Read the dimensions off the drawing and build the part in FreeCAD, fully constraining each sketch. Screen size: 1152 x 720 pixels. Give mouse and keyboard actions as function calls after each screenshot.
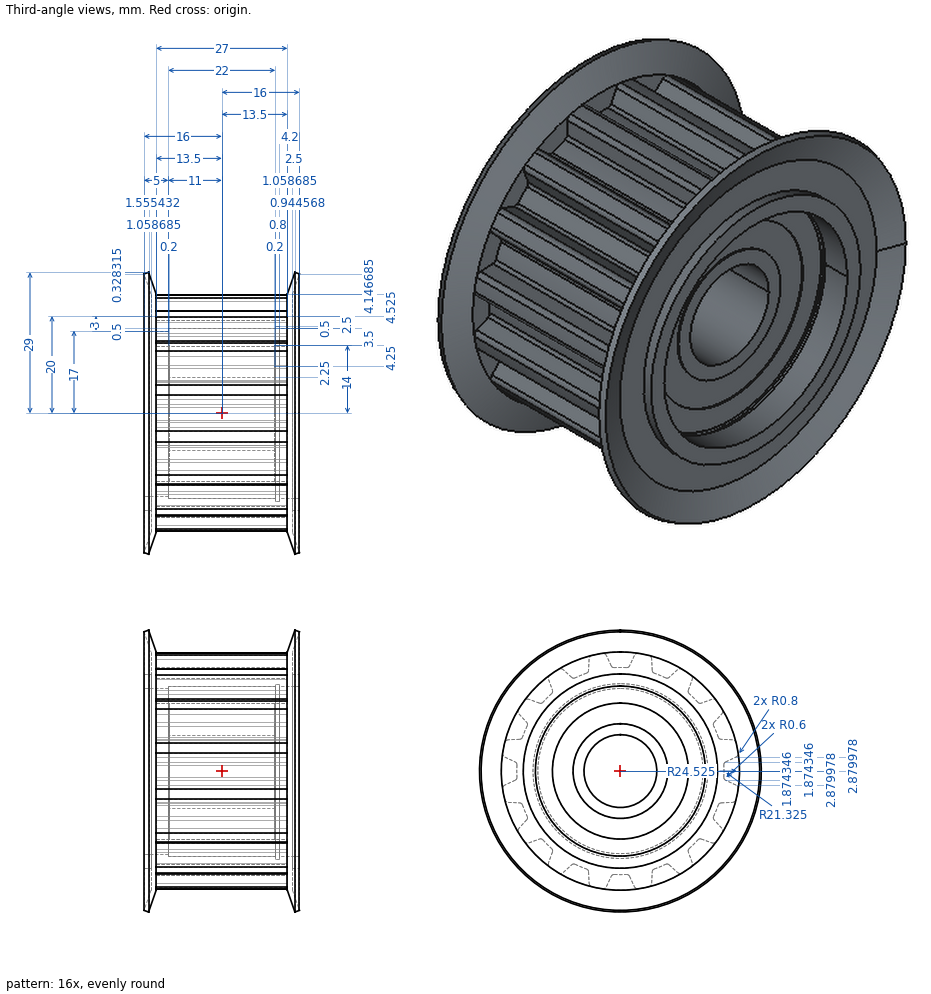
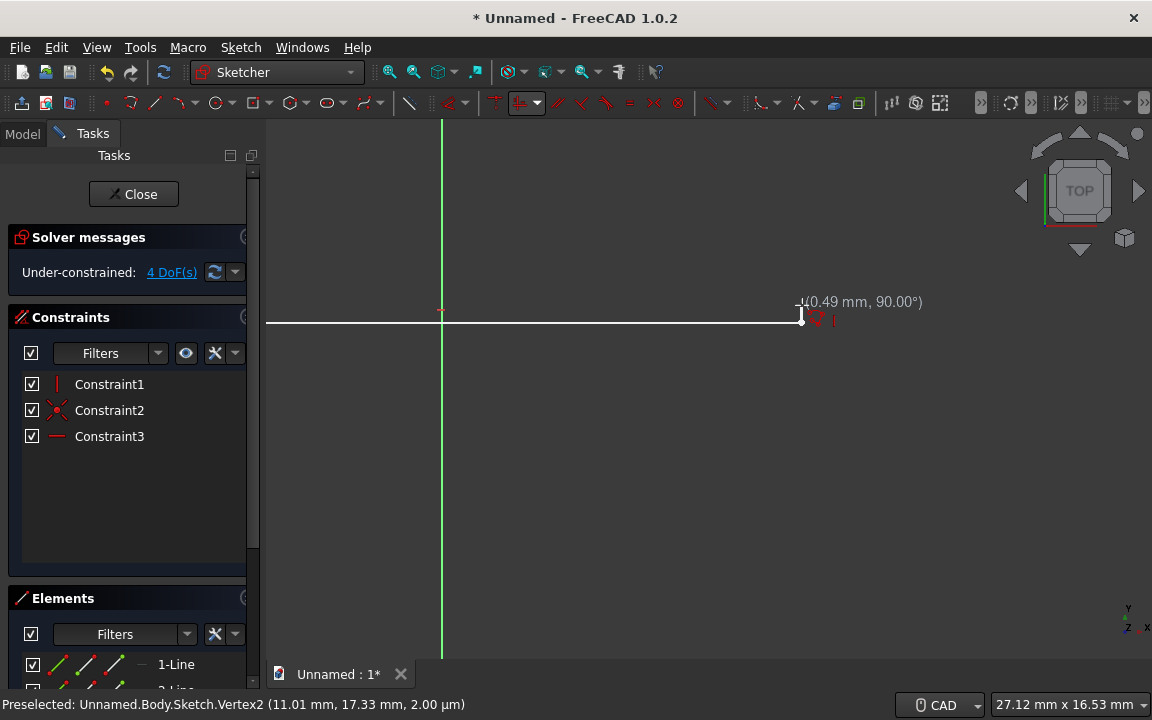
click(801, 305)
click(827, 305)
click(827, 321)
click(964, 321)
click(964, 240)
click(883, 240)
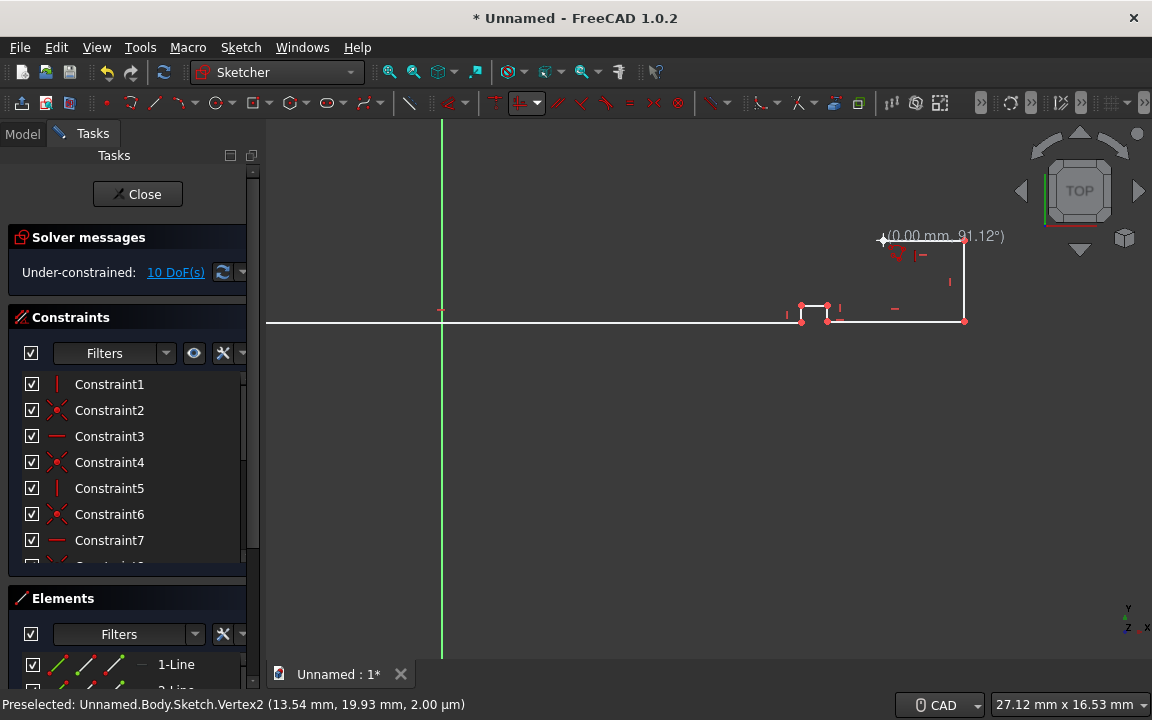
scroll(803, 305, down, 4)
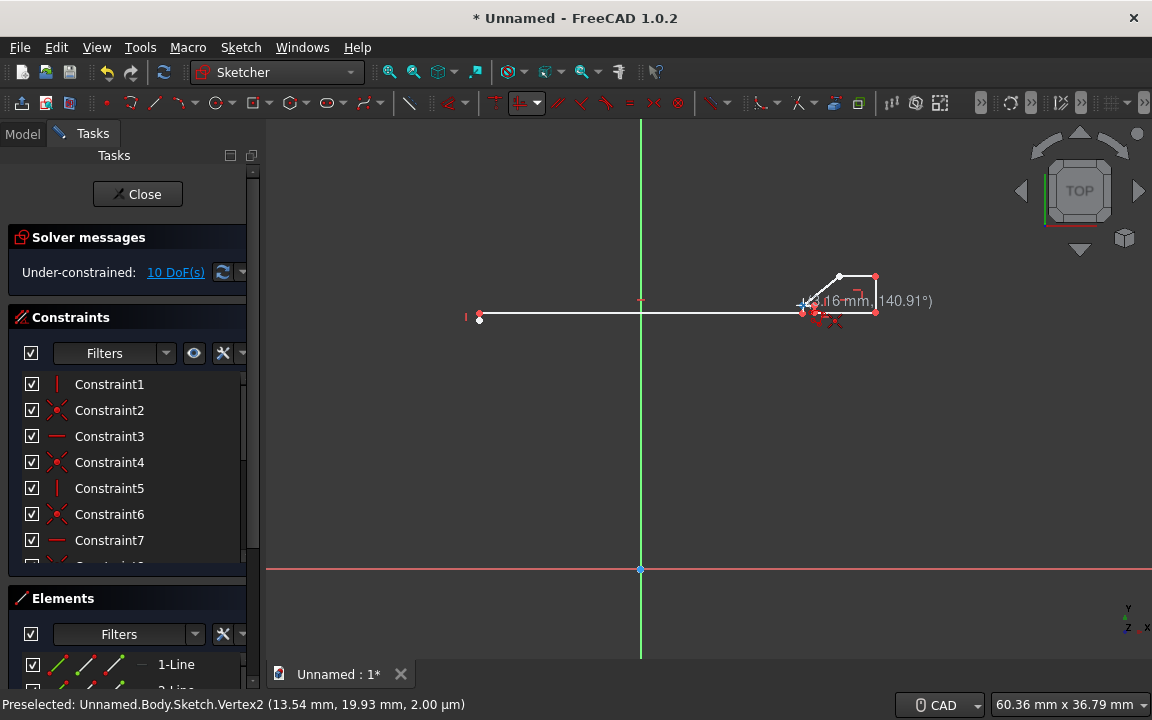
click(839, 209)
click(443, 209)
click(443, 276)
click(406, 276)
click(406, 320)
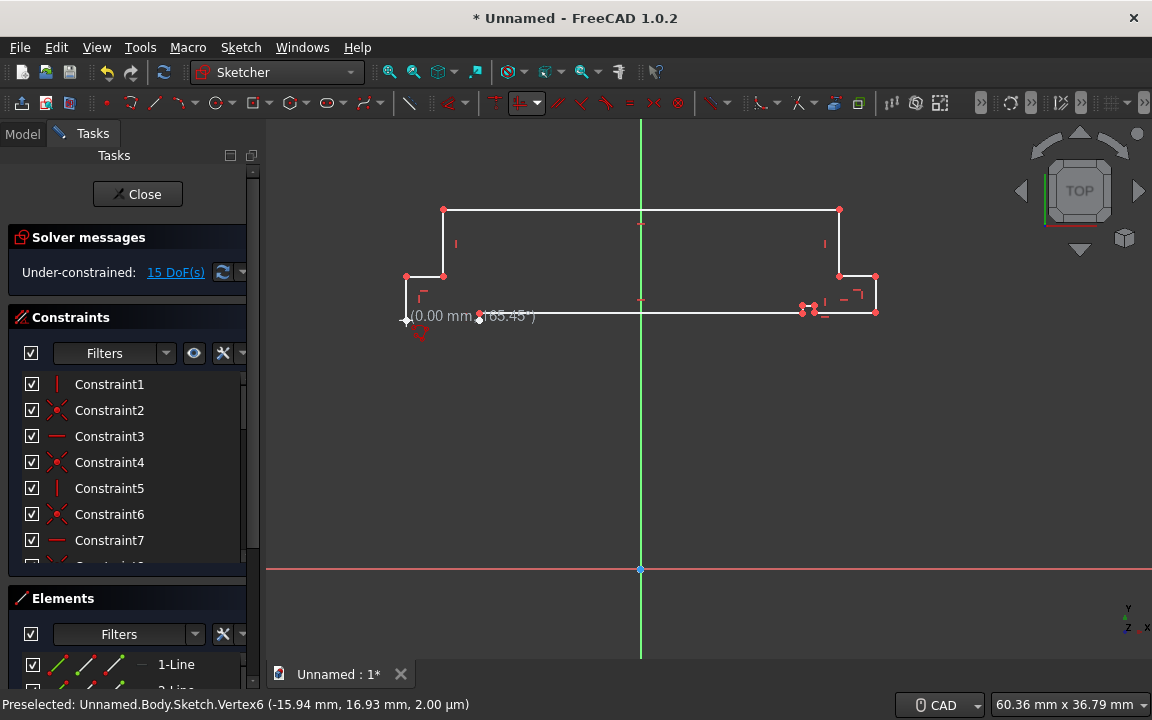
scroll(480, 320, up, 8)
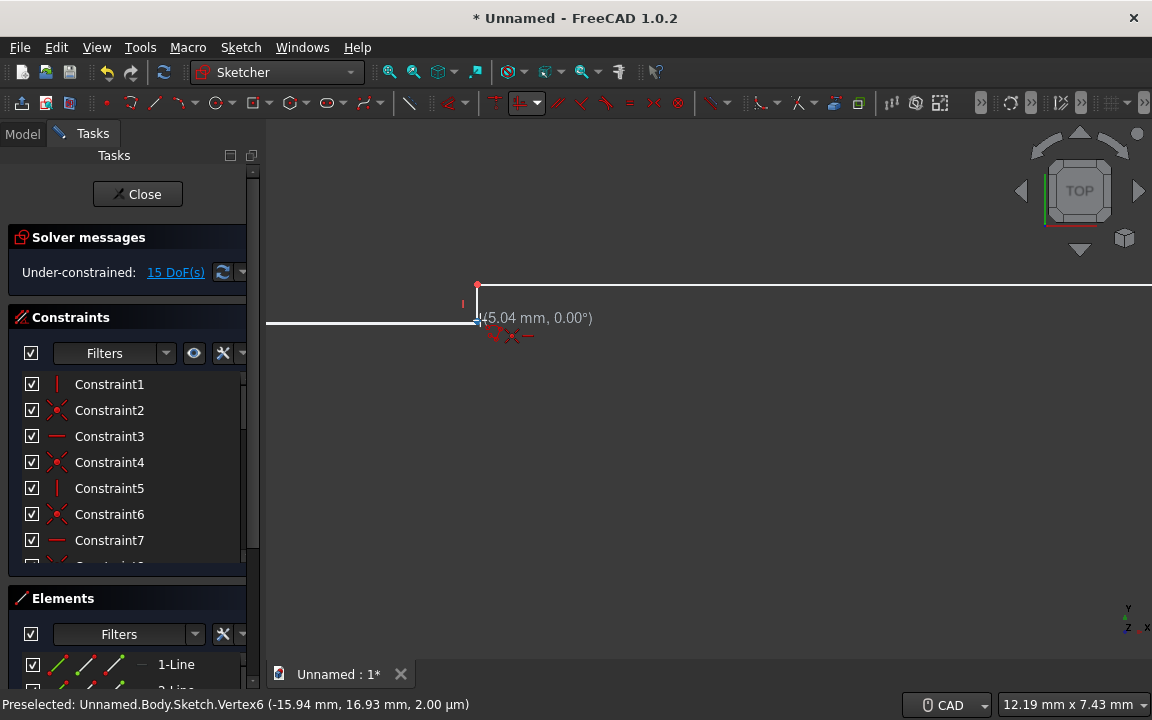
click(477, 321)
key(Escape)
key(Escape)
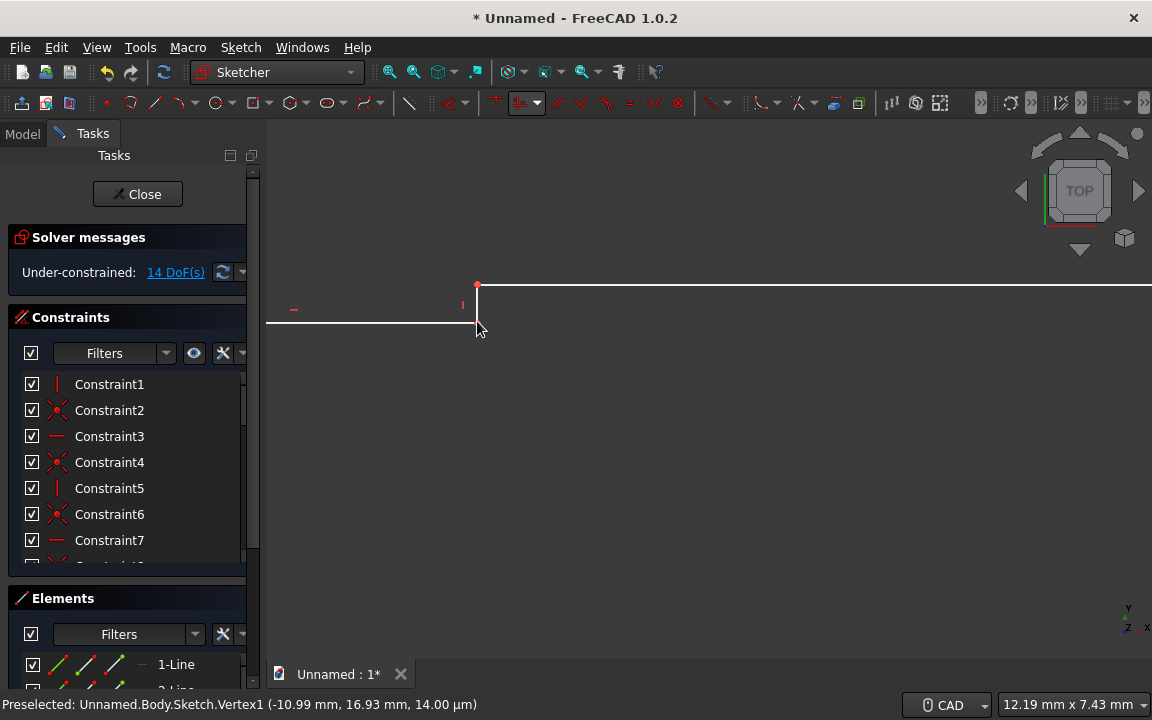
scroll(480, 320, down, 8)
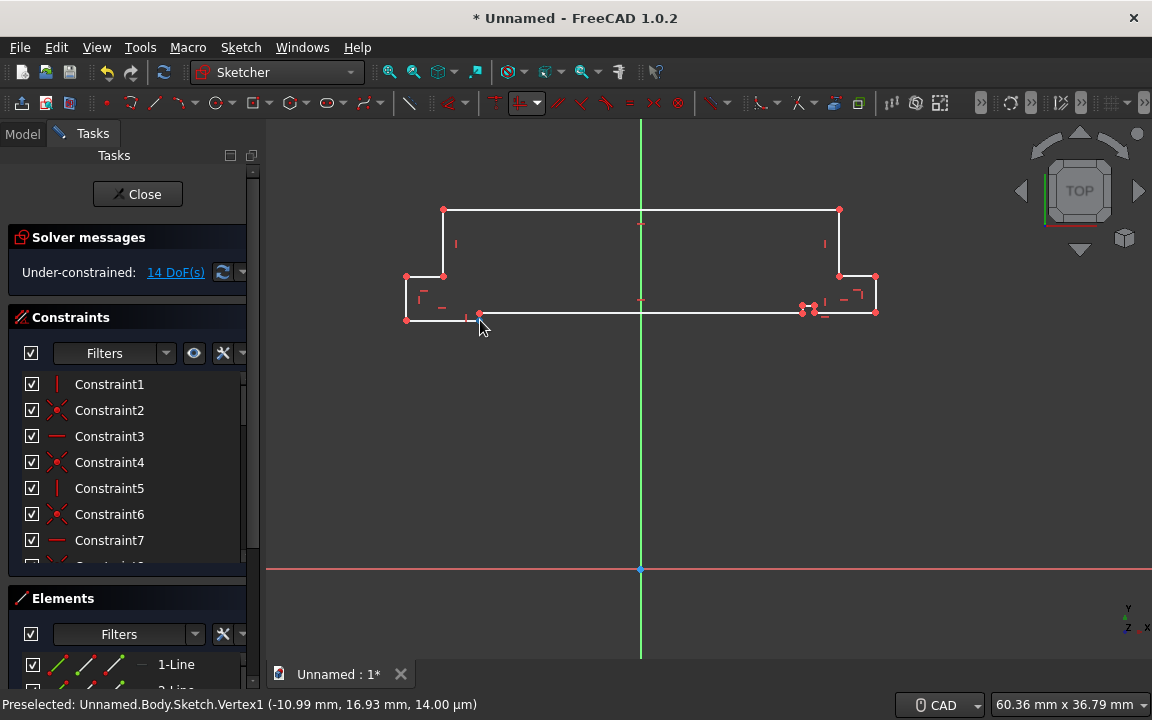
click(406, 290)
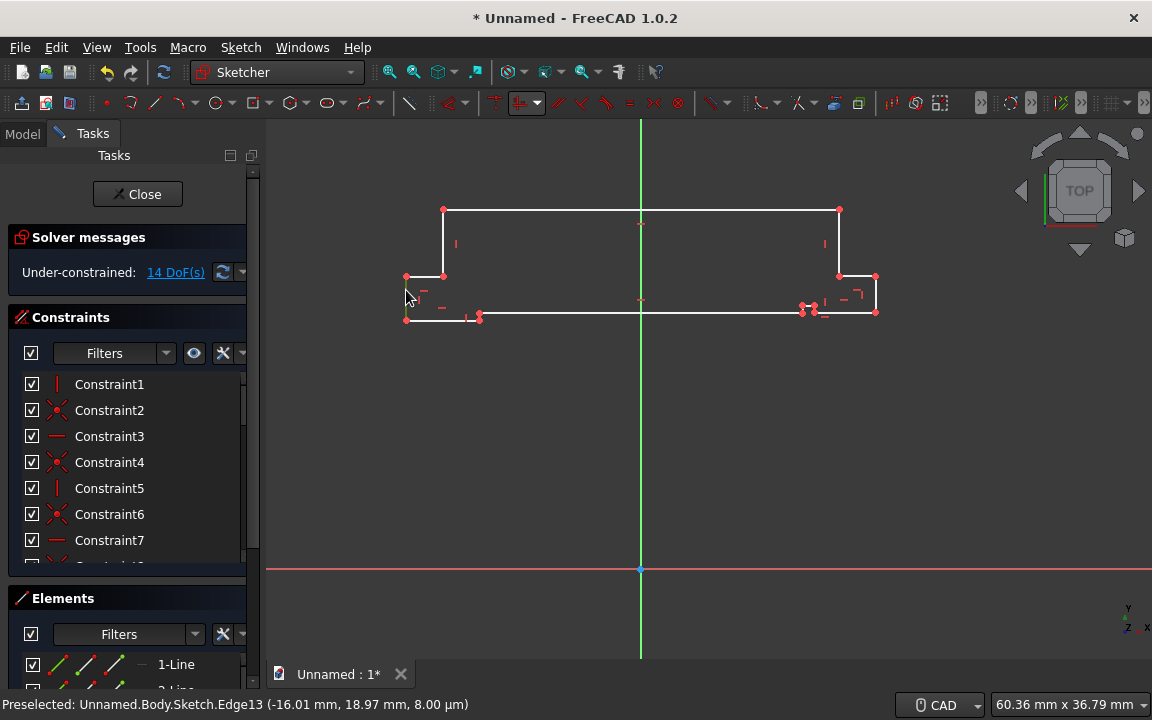
key(i)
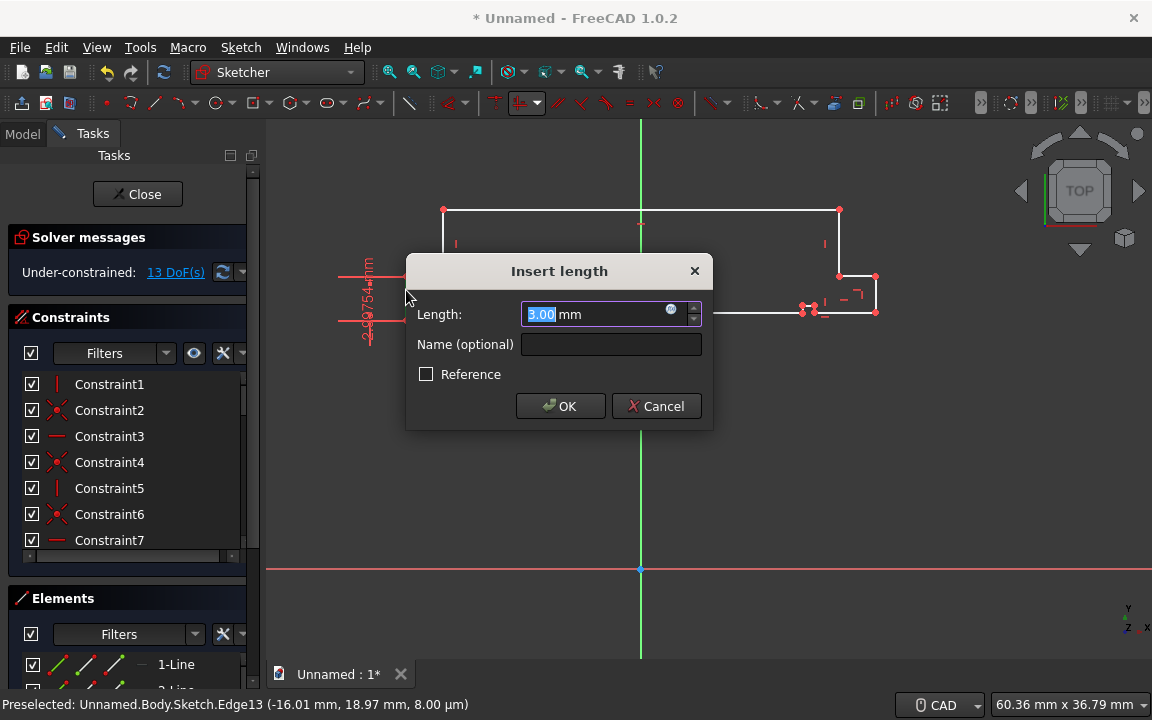
text(3)
key(Return)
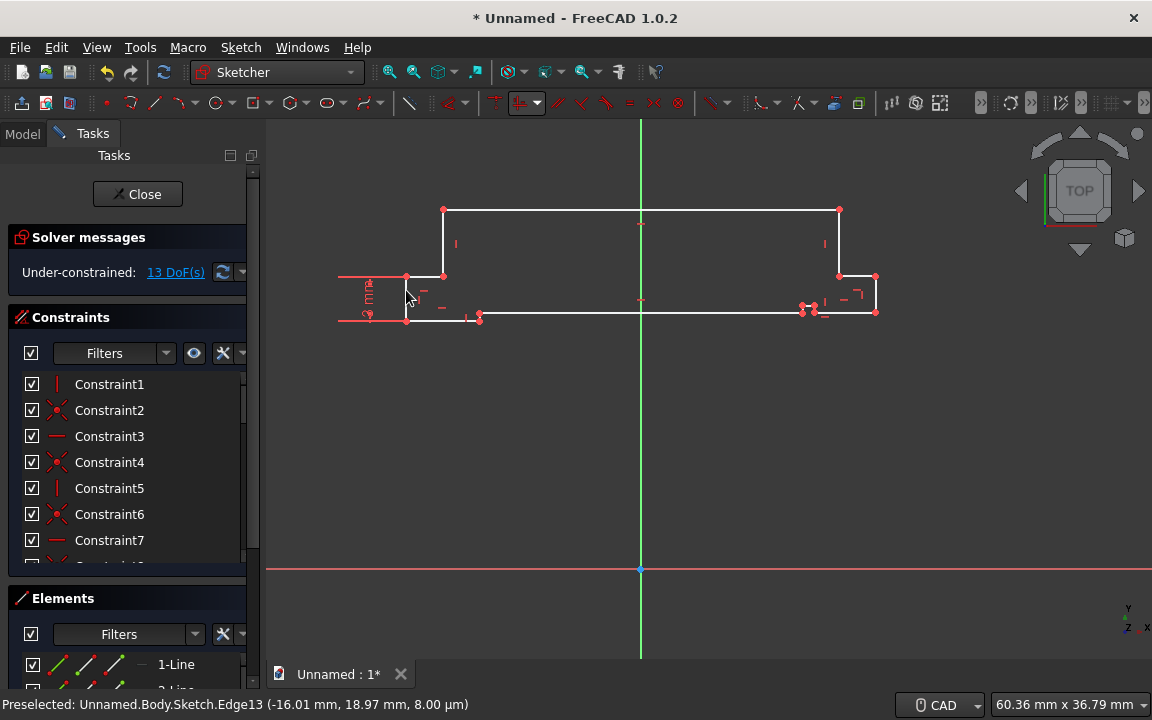
click(428, 321)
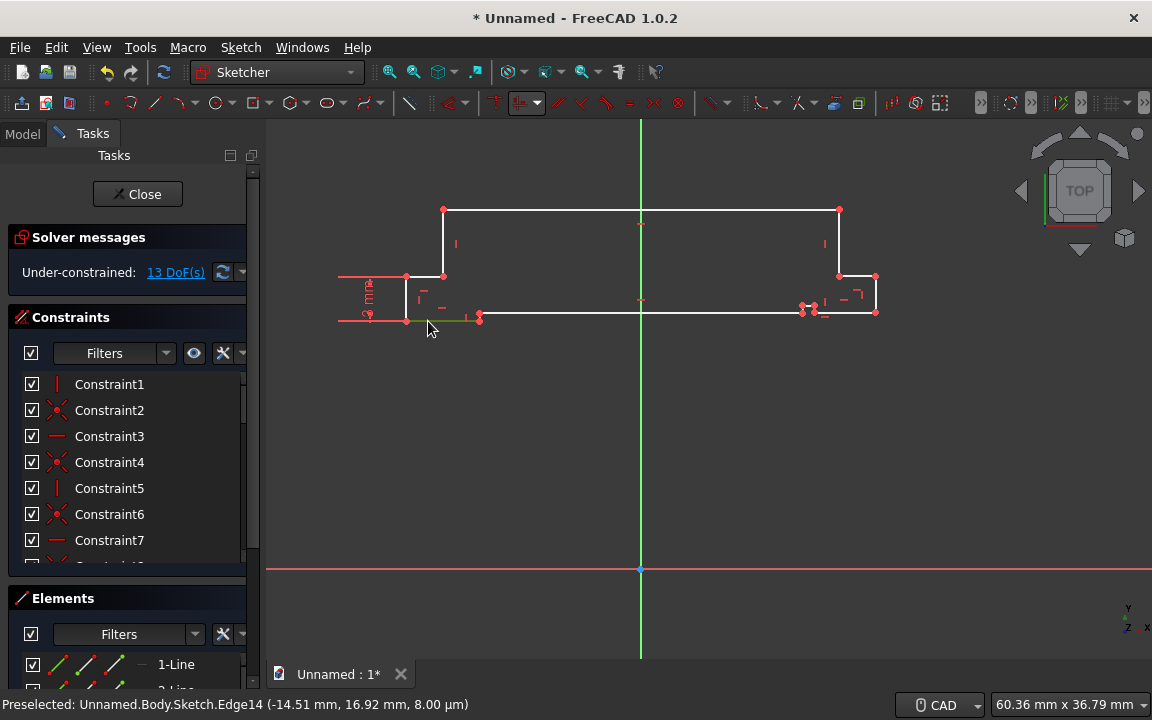
click(468, 104)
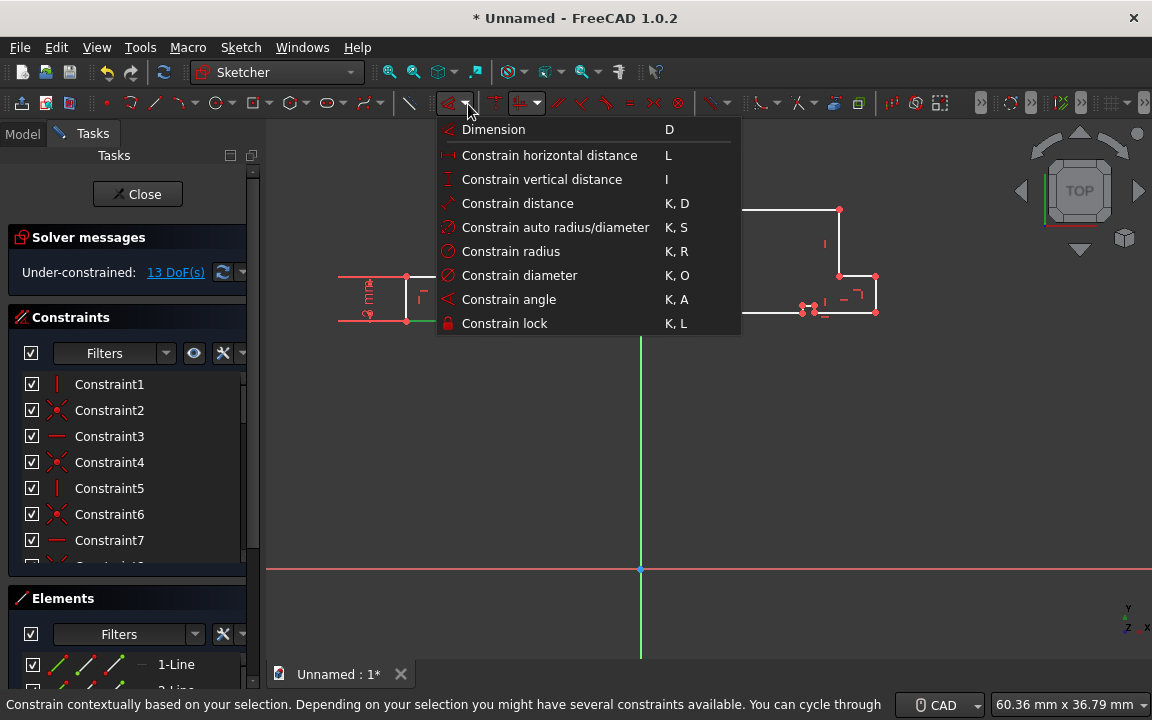
click(589, 155)